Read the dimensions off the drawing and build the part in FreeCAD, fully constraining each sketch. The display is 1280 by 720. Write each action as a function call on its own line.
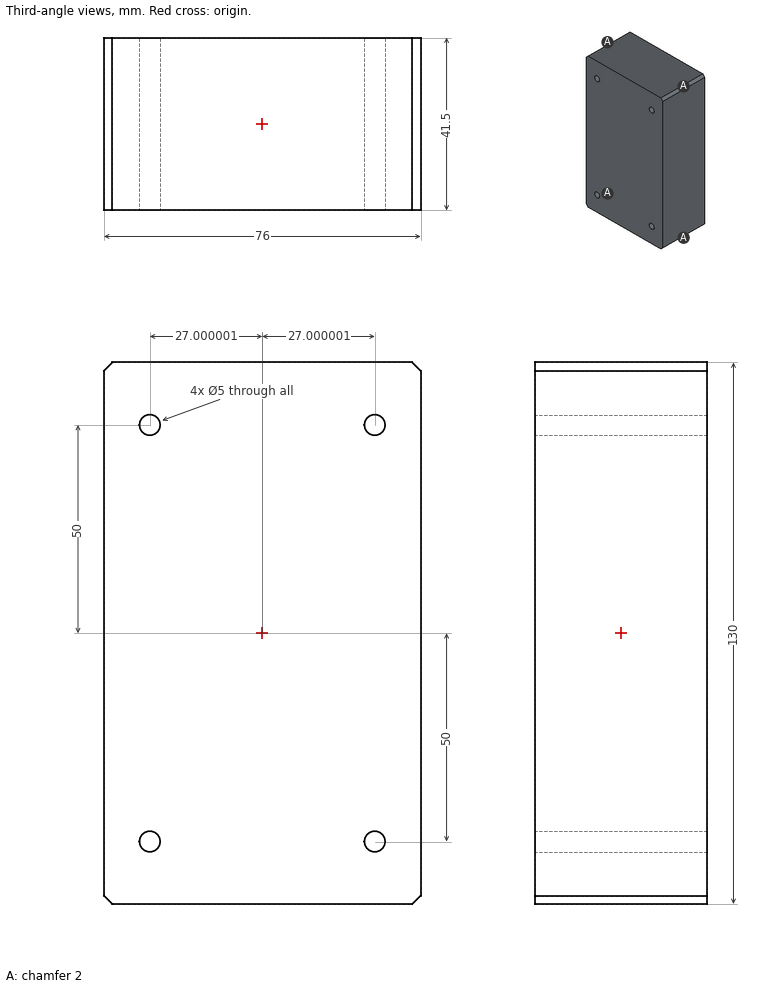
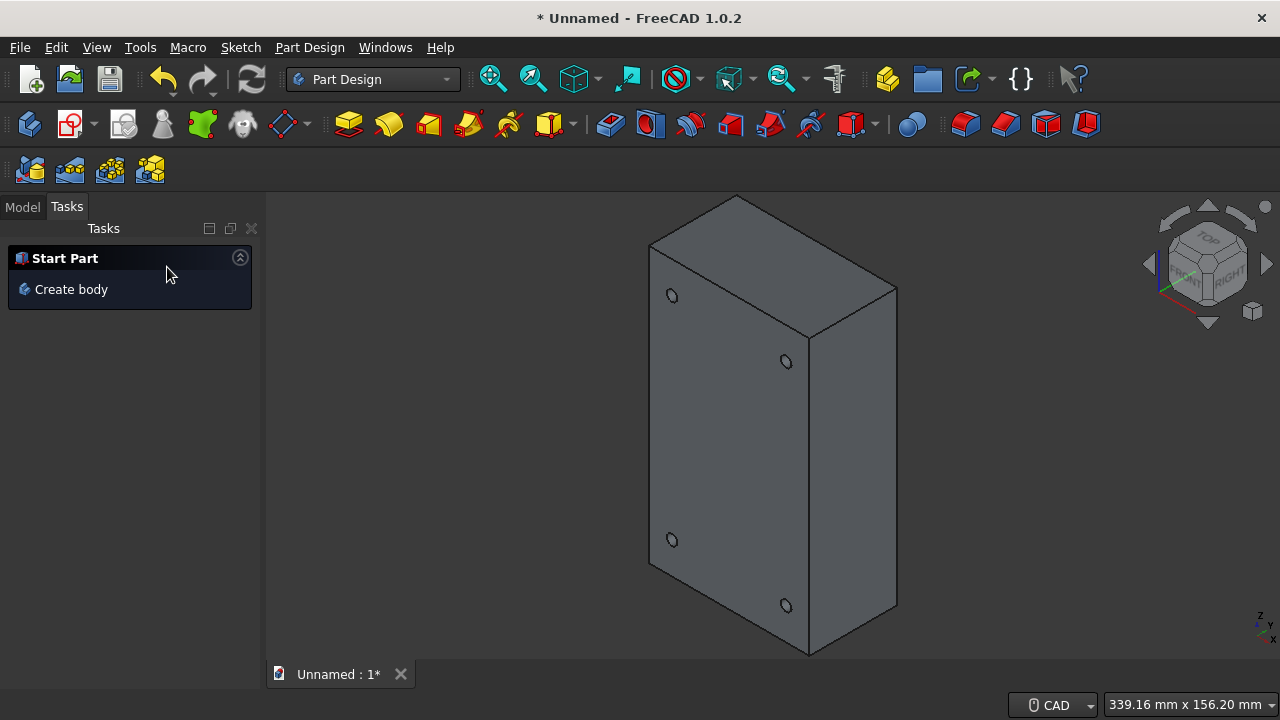
click(853, 312)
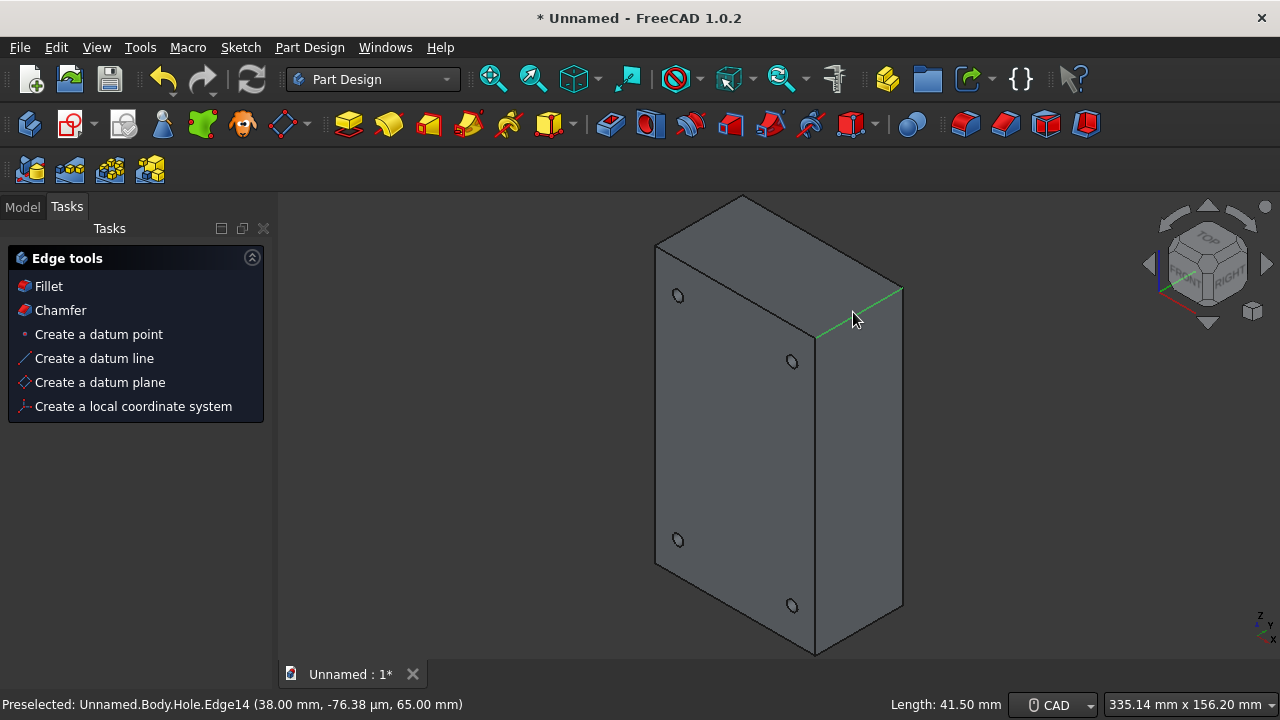
key(2)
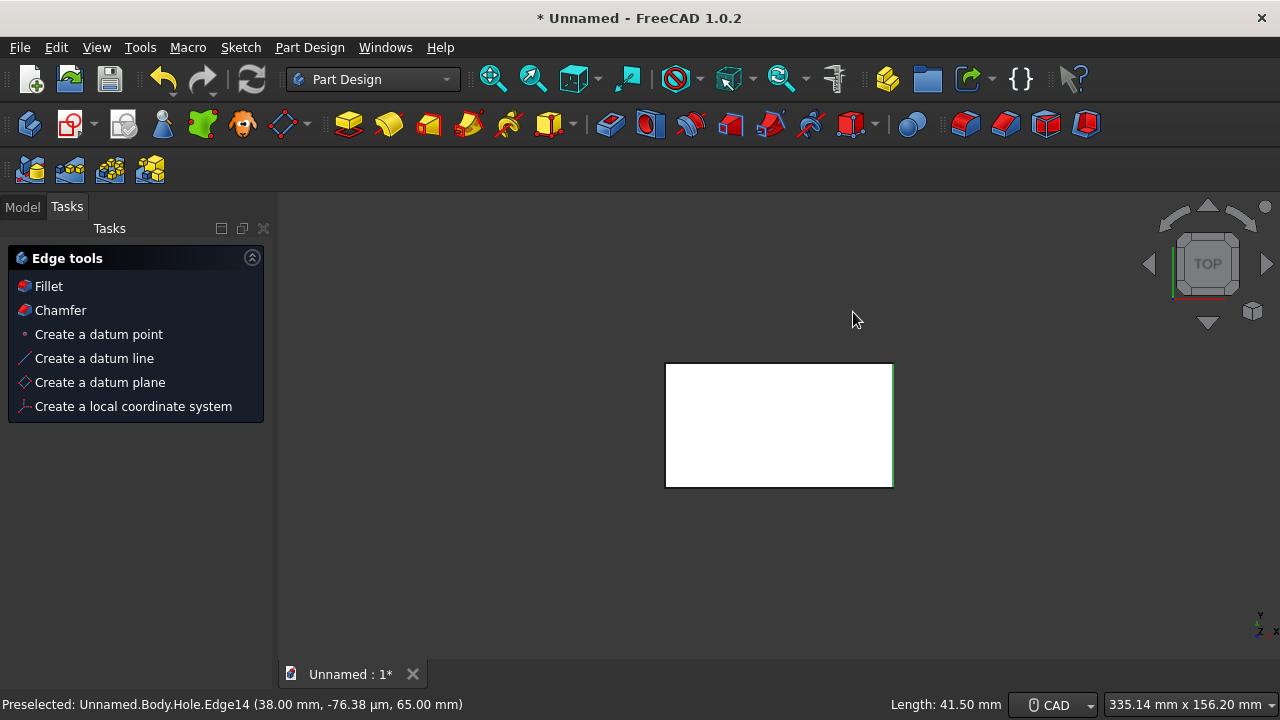
click(494, 80)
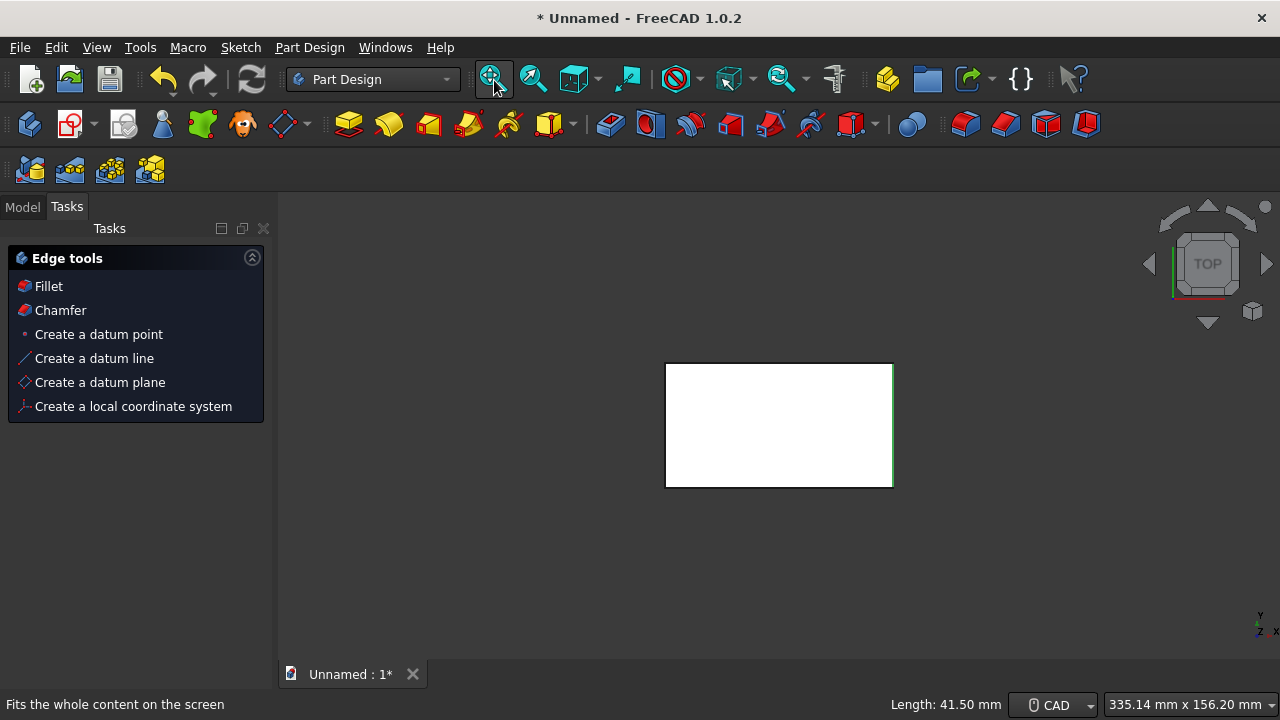
click(665, 424, ctrl)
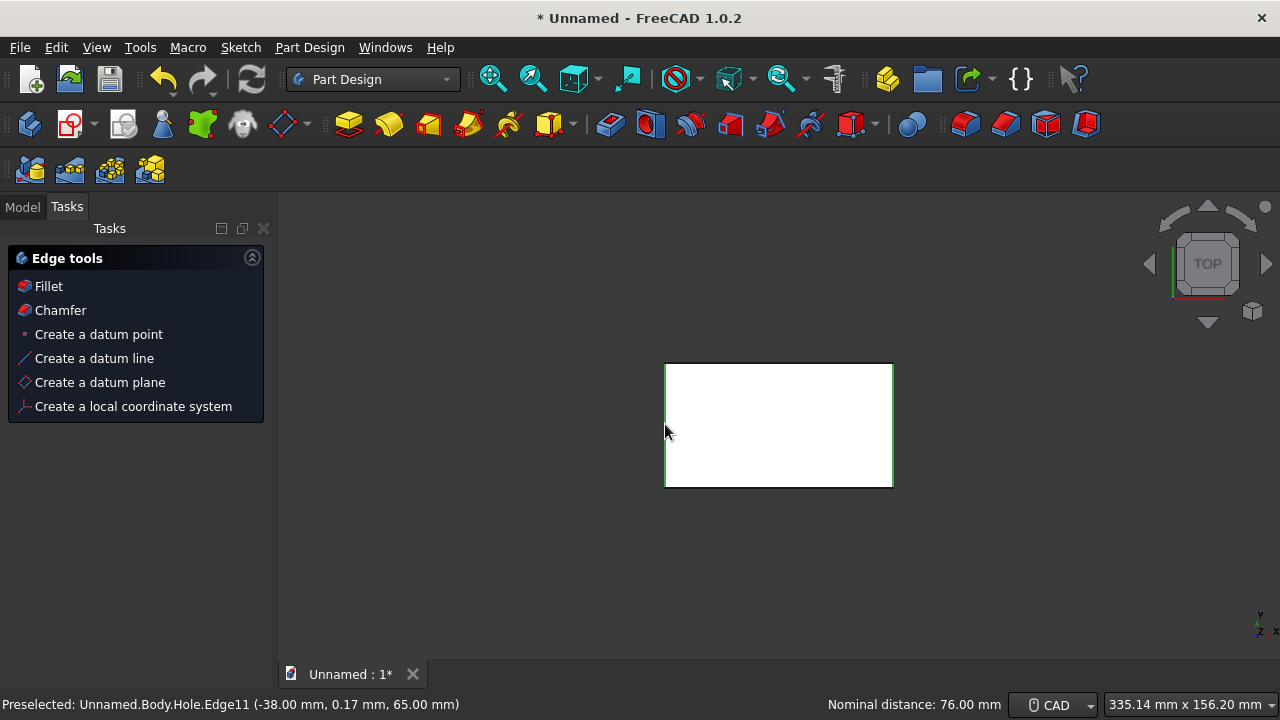
key(1)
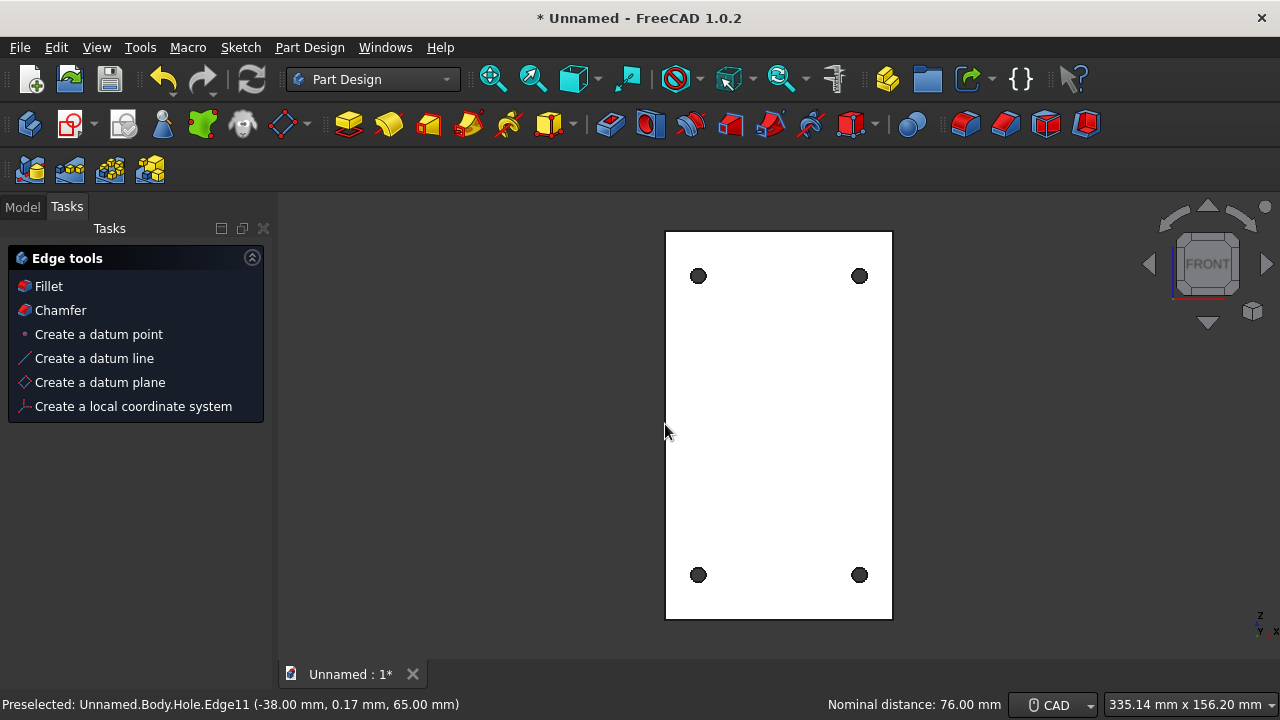
key(3)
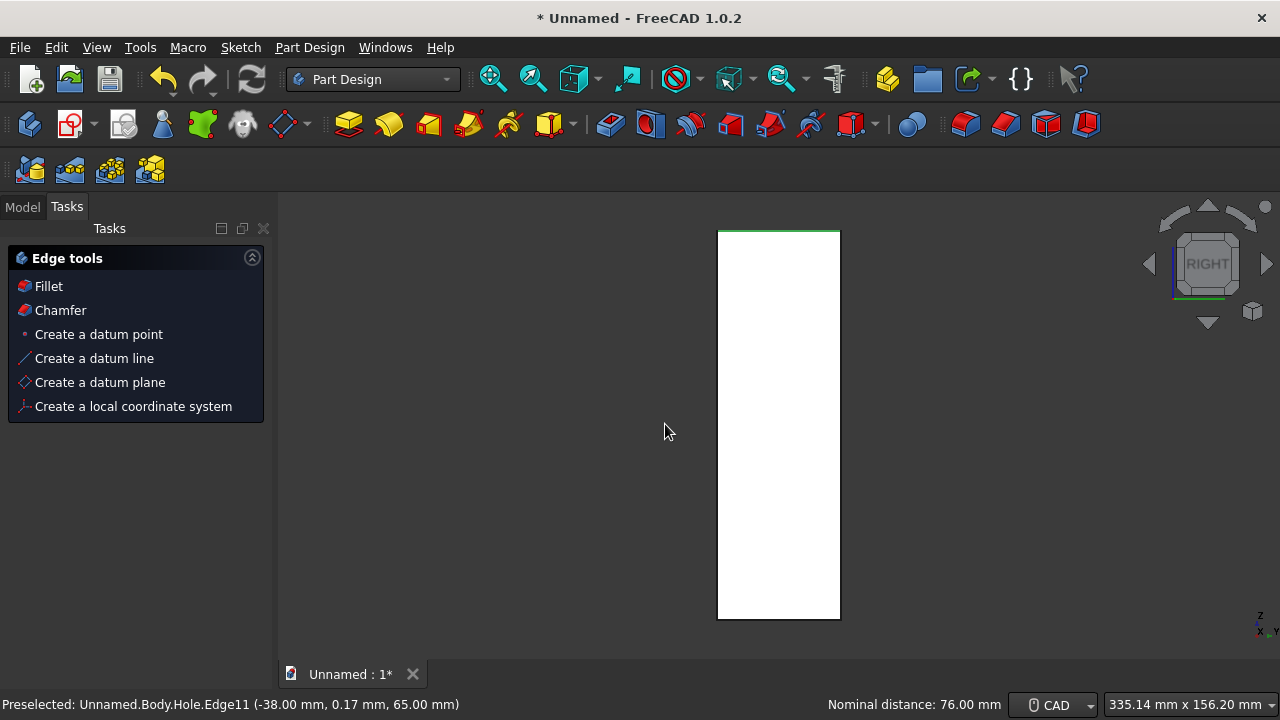
click(779, 619, ctrl)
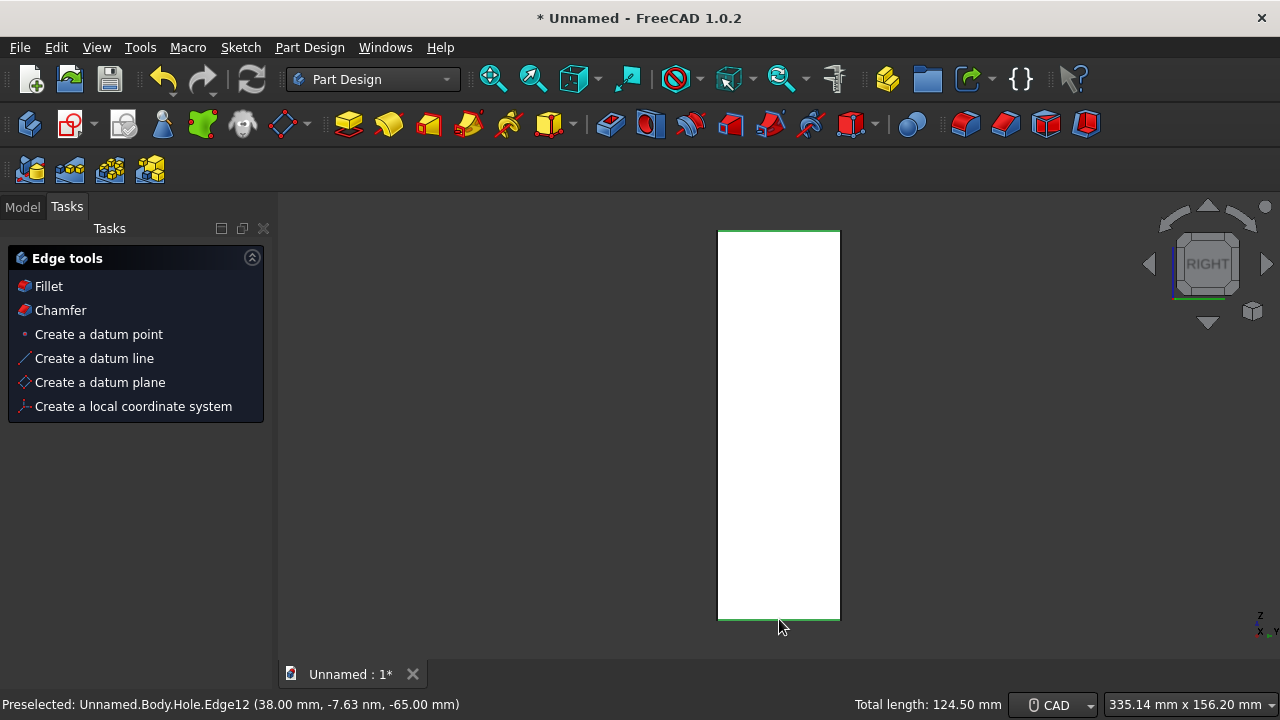
key(5)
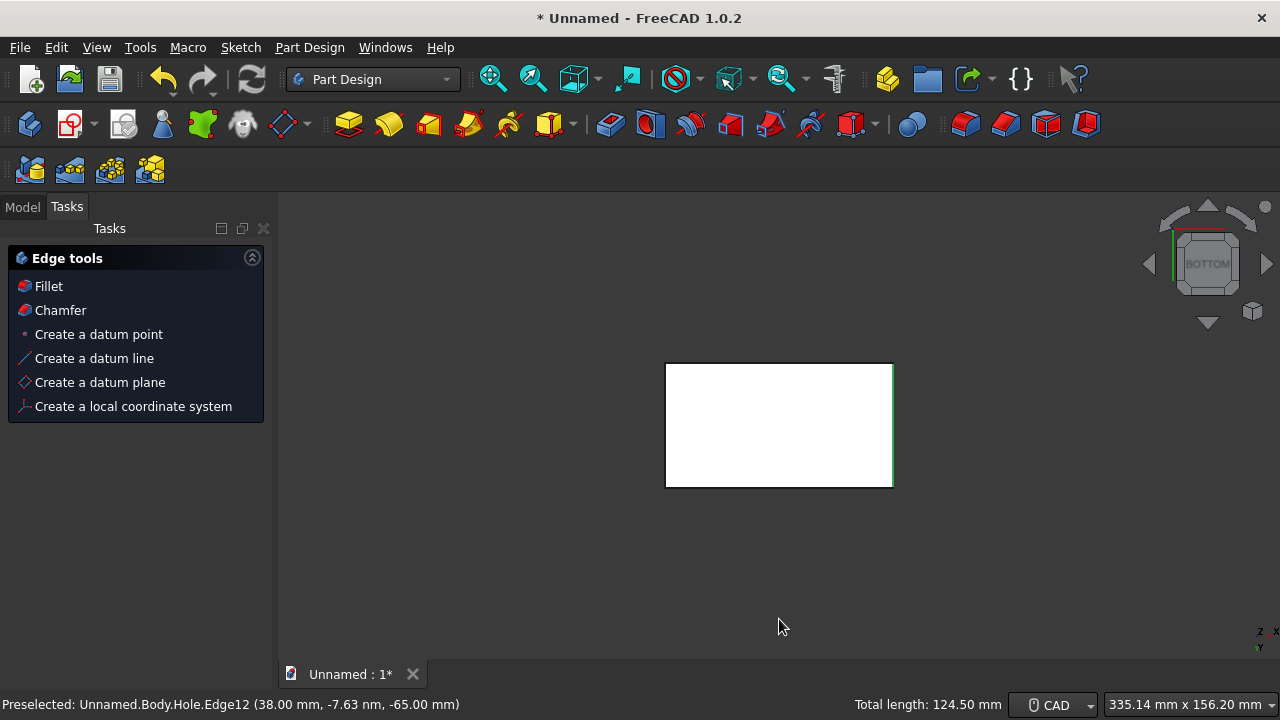
click(494, 80)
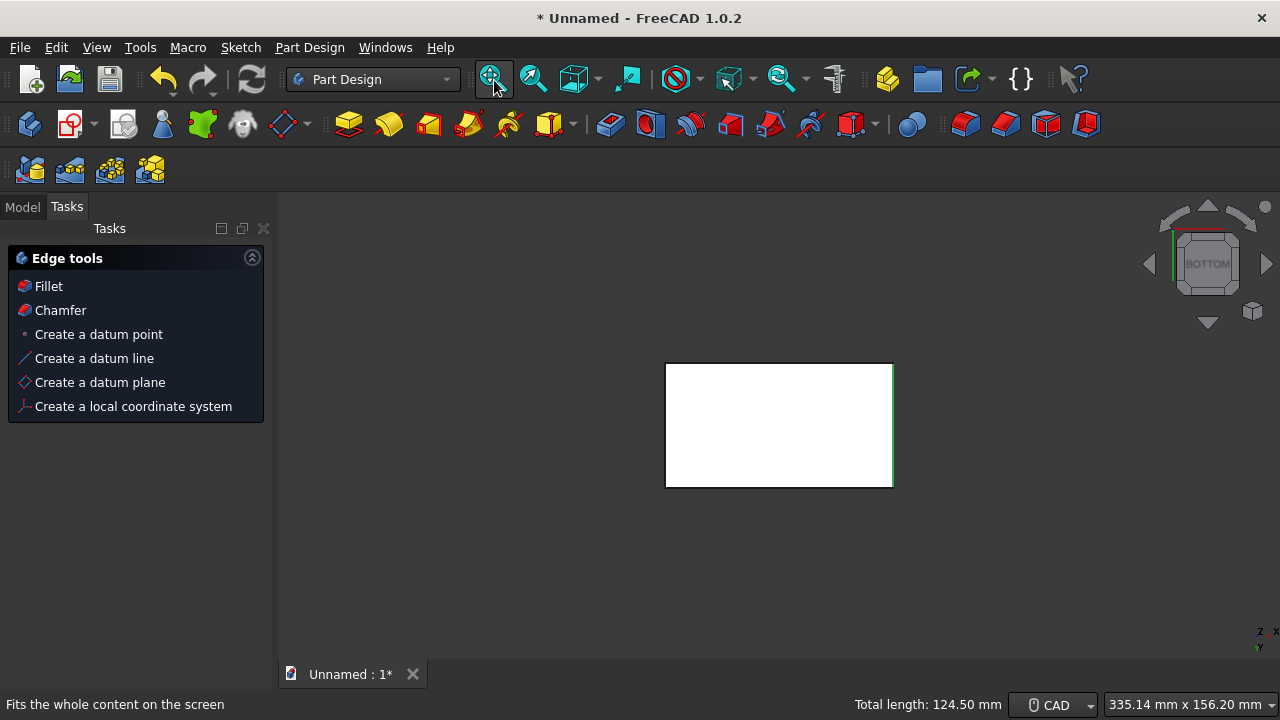
click(665, 424, ctrl)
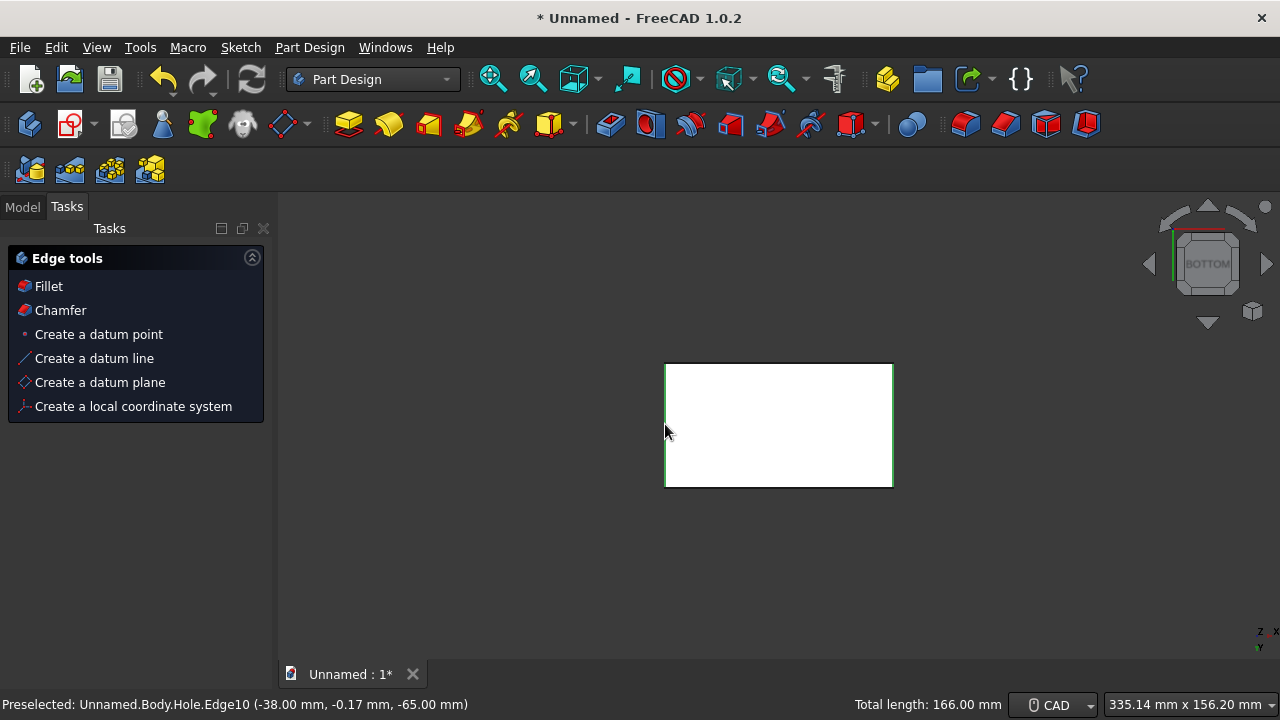
click(1006, 124)